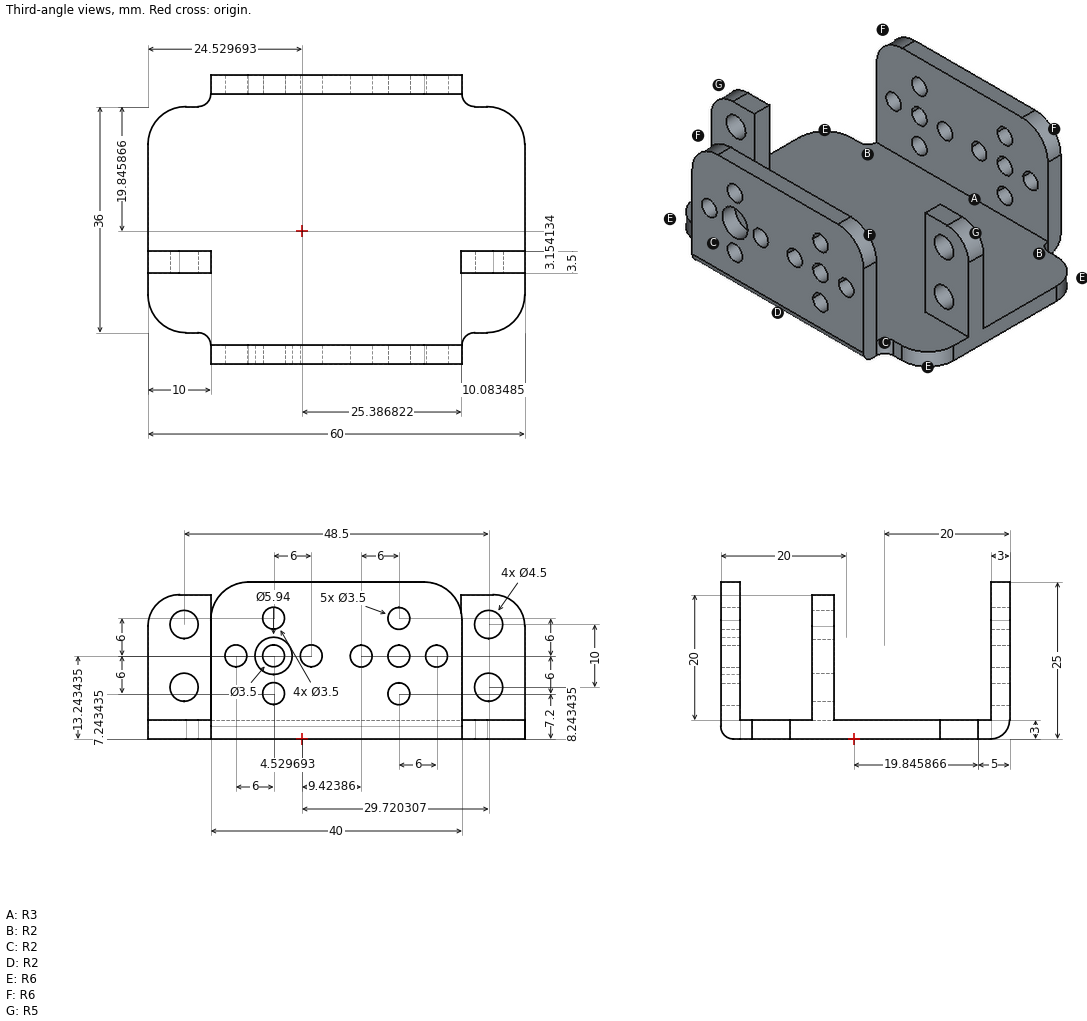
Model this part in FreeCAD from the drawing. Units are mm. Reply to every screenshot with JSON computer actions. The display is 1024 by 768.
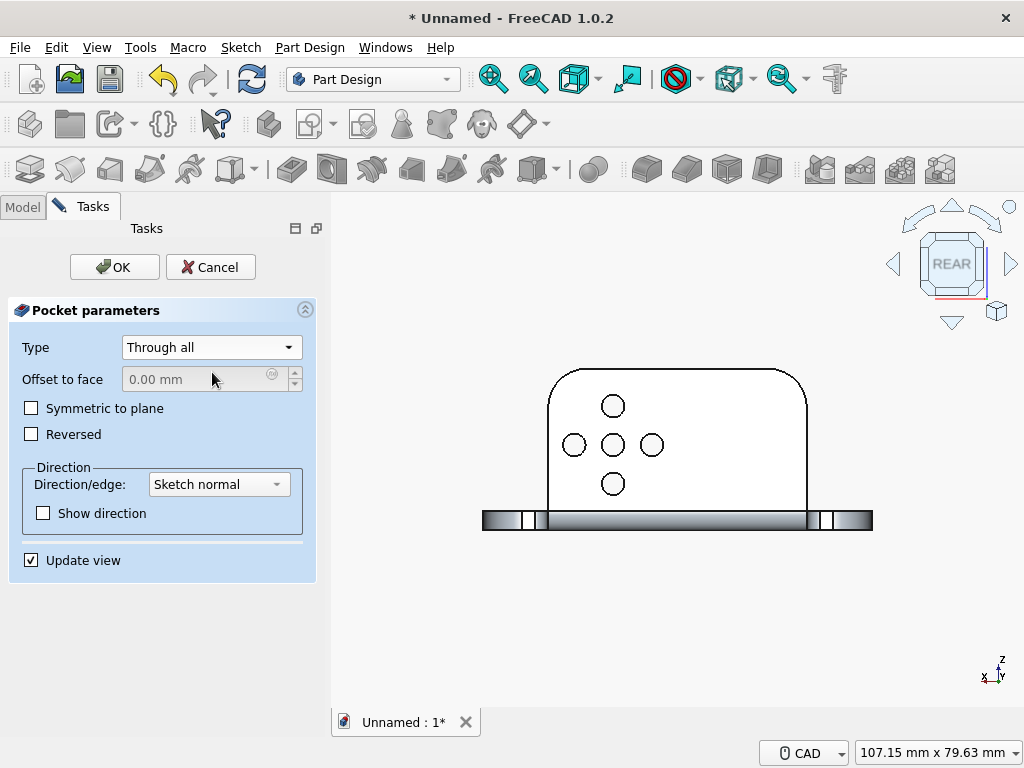
{"action": "left_click", "coordinate": [115, 267]}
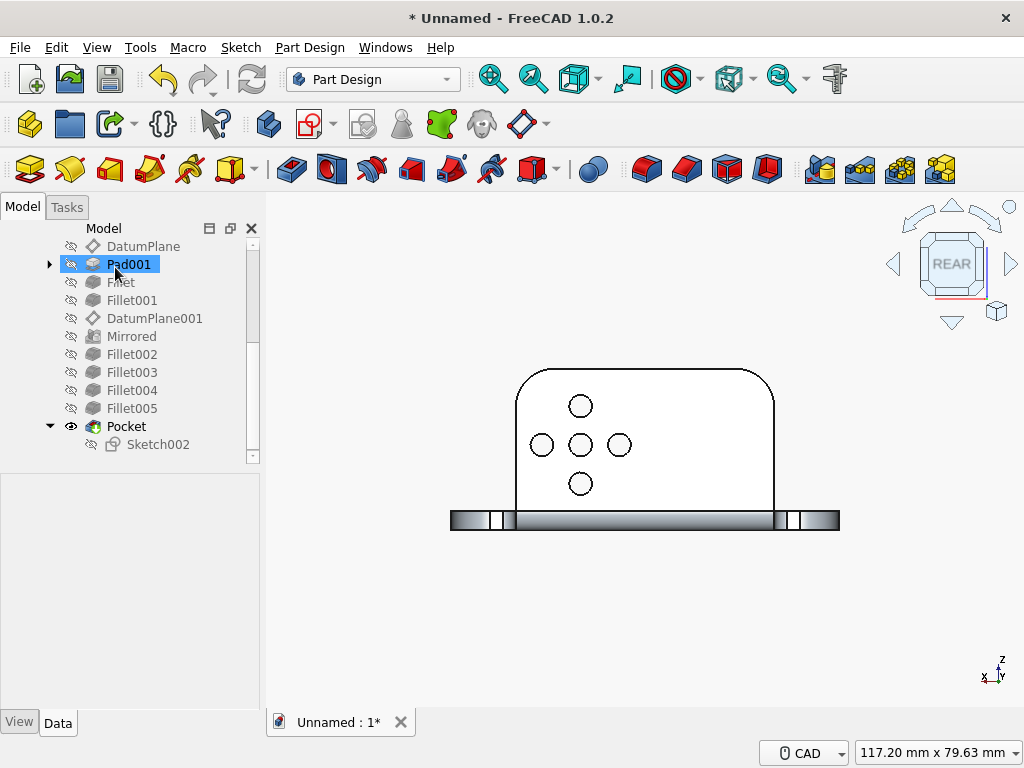
{"action": "key", "text": "0"}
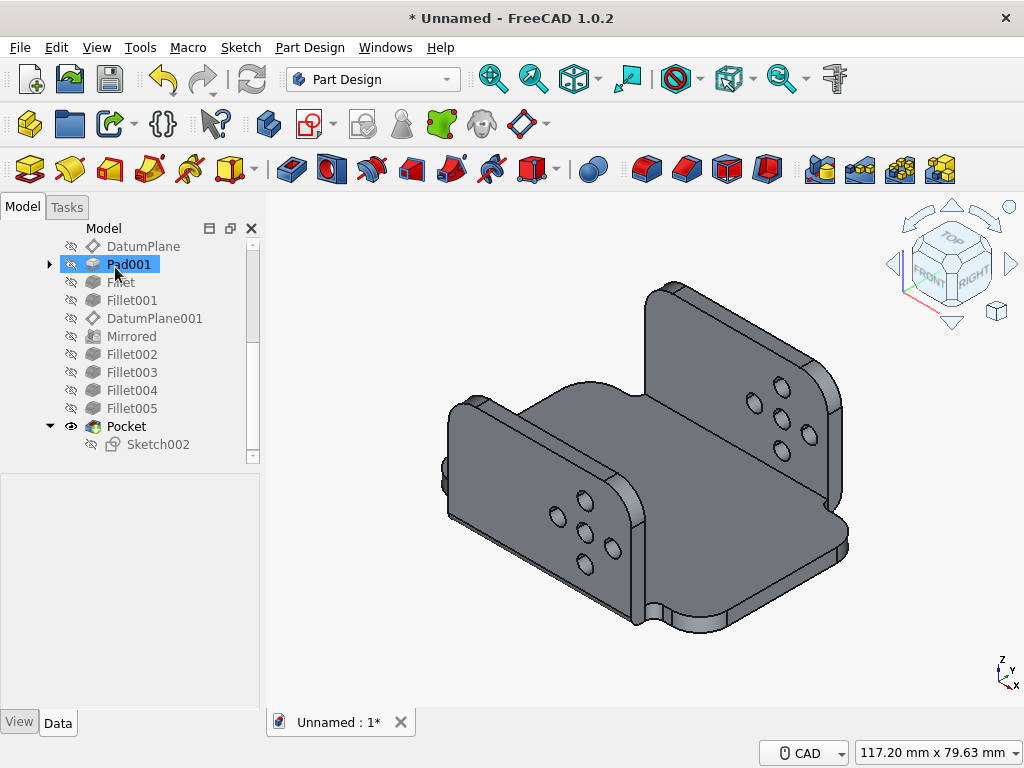
{"action": "left_click", "coordinate": [684, 521]}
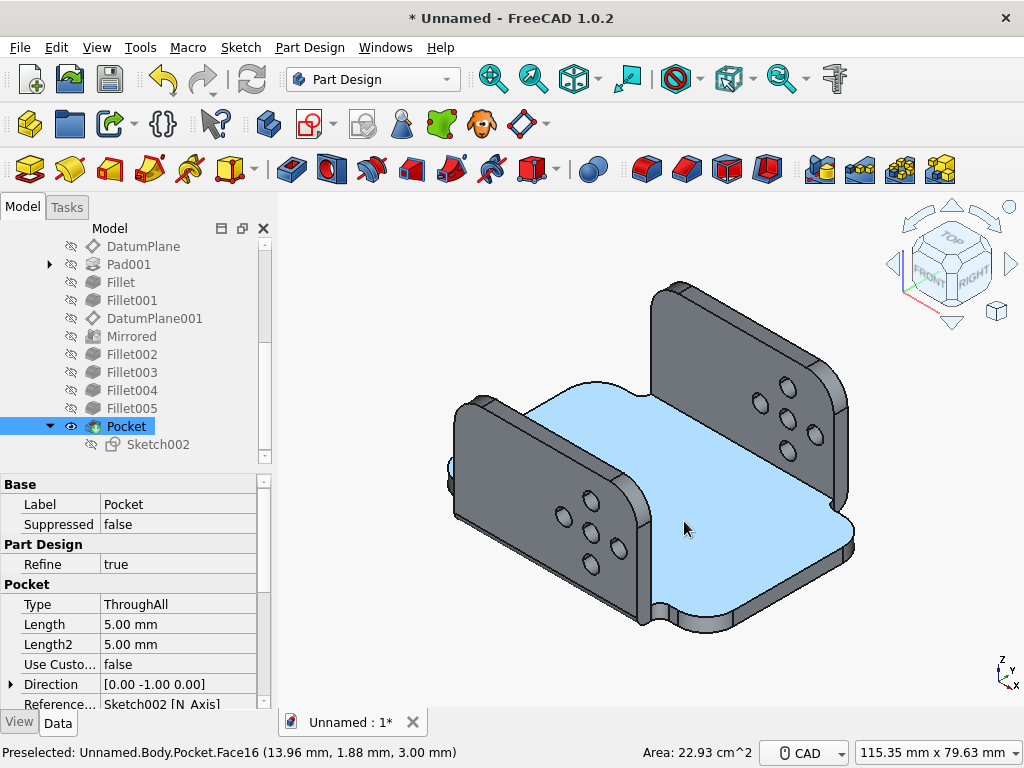
{"action": "left_click", "coordinate": [310, 124]}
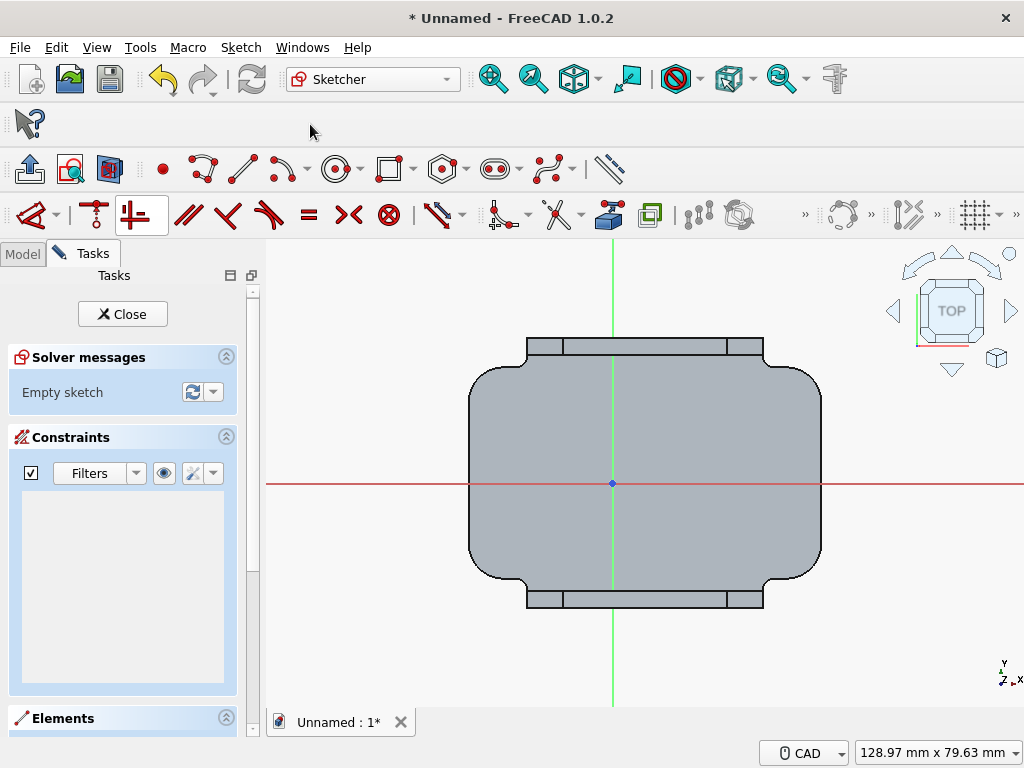
{"action": "left_click", "coordinate": [110, 170]}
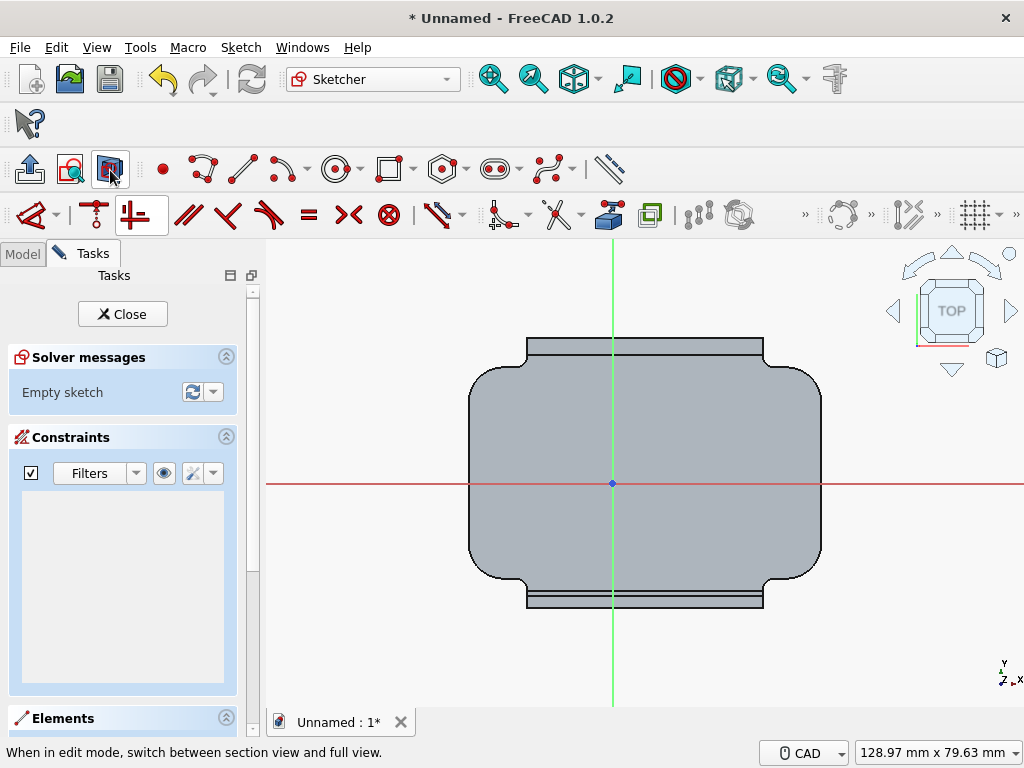
{"action": "left_click", "coordinate": [390, 170]}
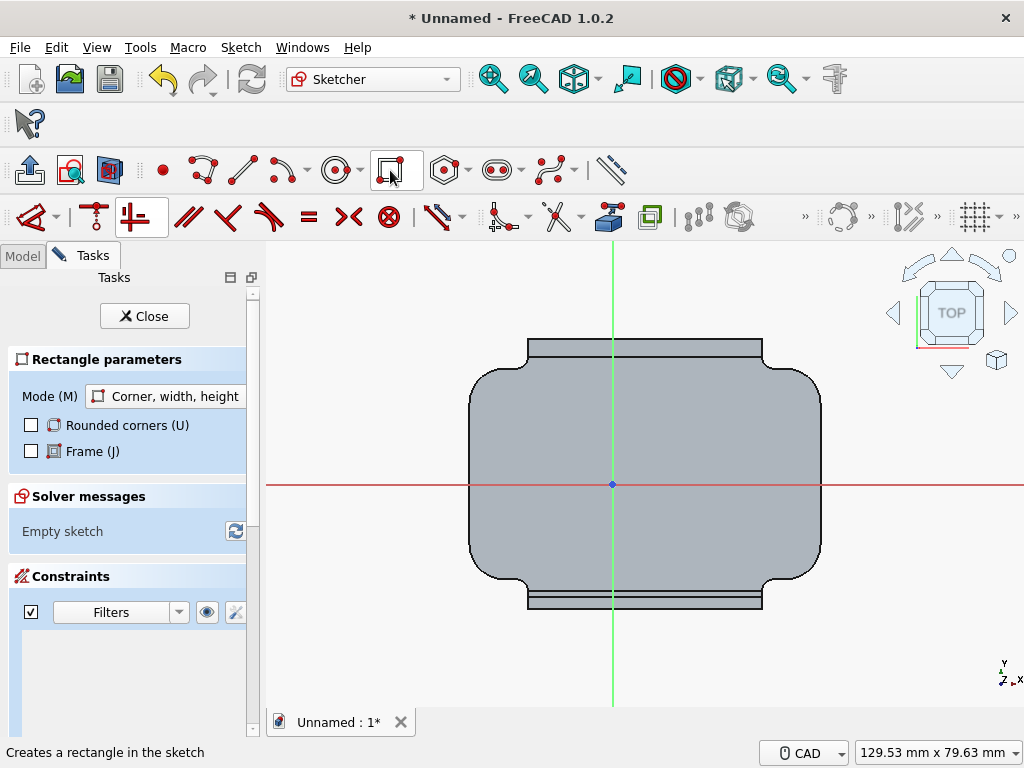
{"action": "left_click", "coordinate": [762, 503]}
{"action": "left_click", "coordinate": [821, 524]}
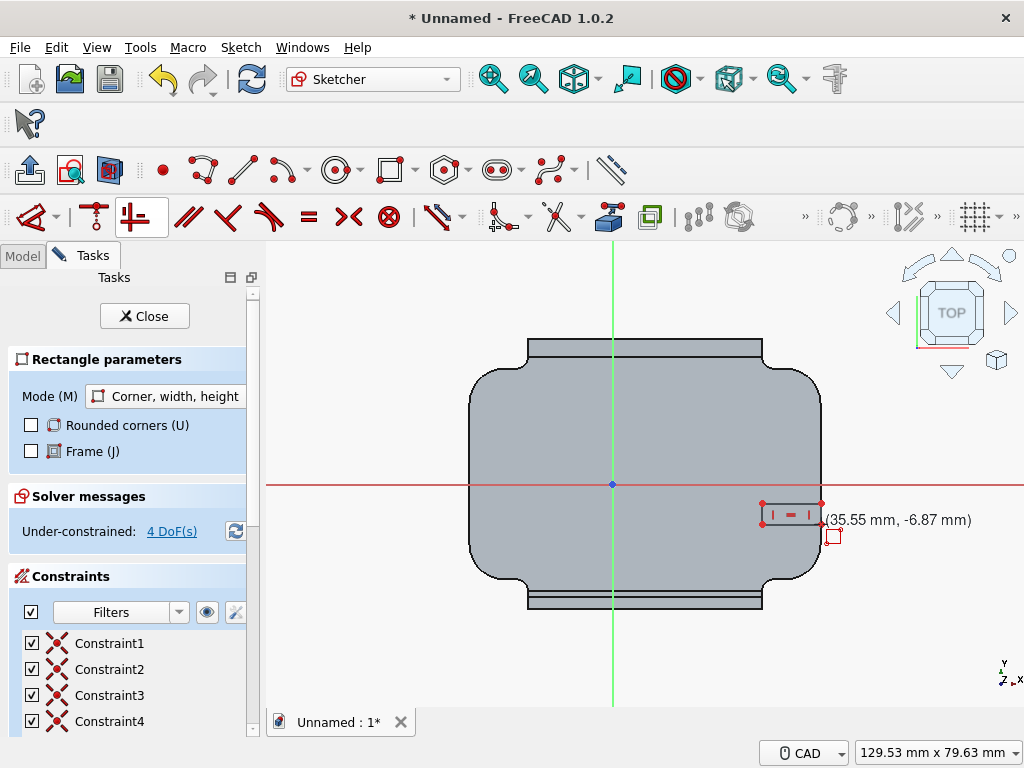
{"action": "left_click", "coordinate": [469, 503]}
{"action": "left_click", "coordinate": [528, 524]}
{"action": "key", "text": "Escape"}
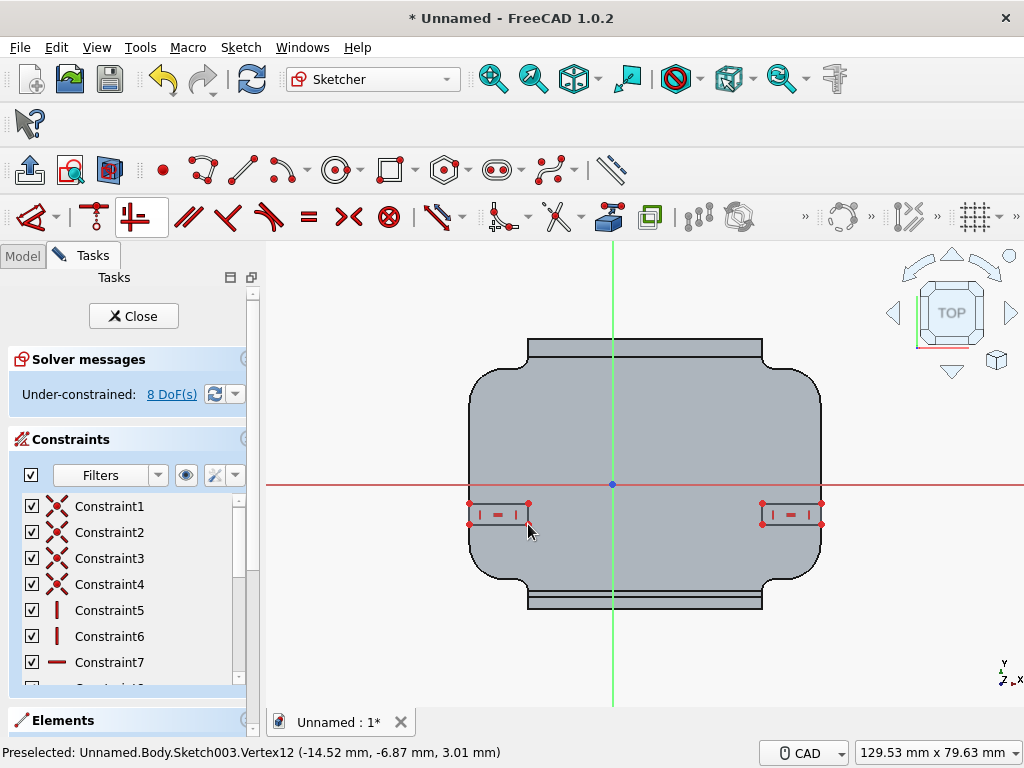
{"action": "left_click", "coordinate": [32, 218]}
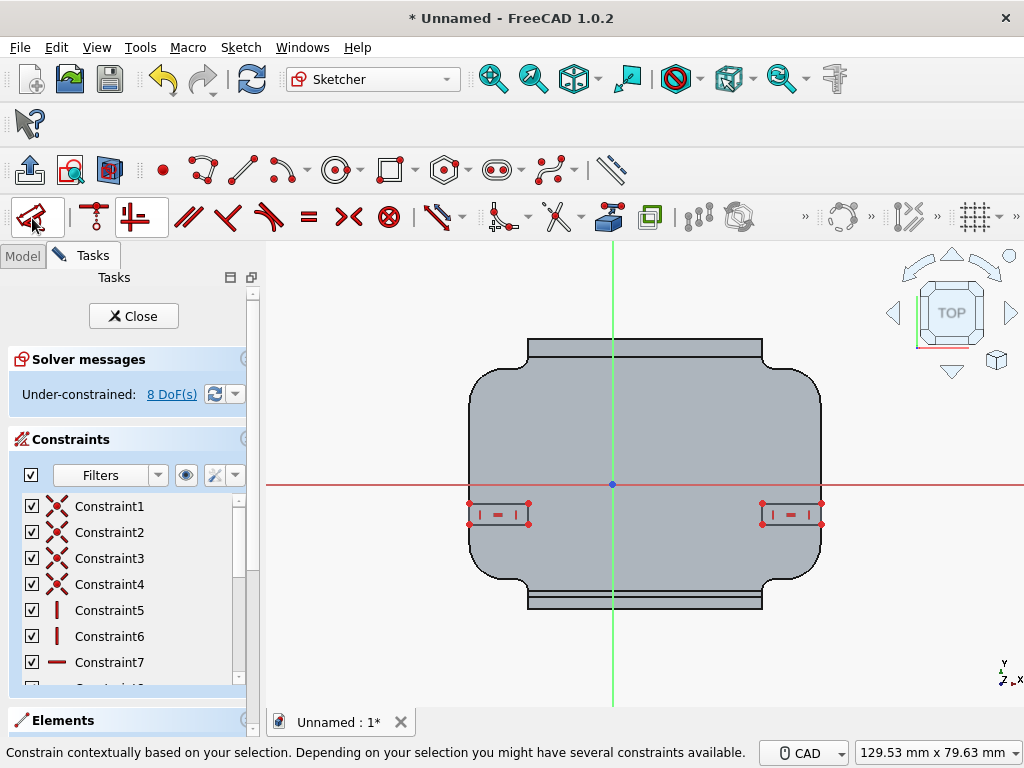
{"action": "left_click", "coordinate": [487, 525]}
{"action": "left_click", "coordinate": [499, 559]}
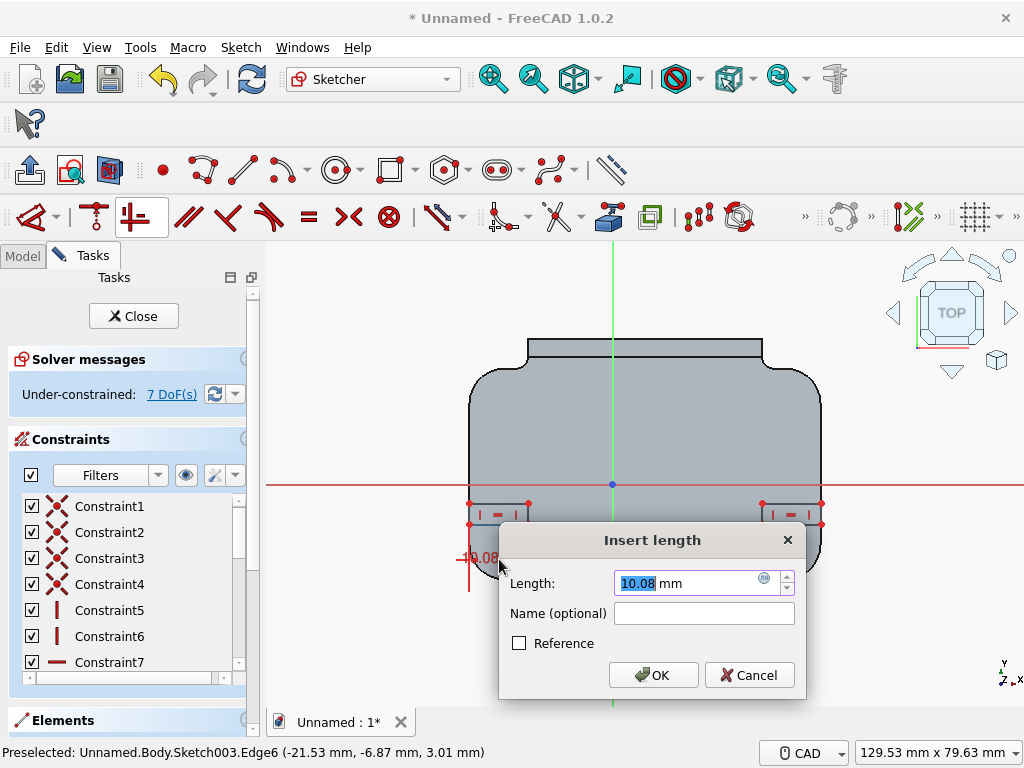
{"action": "type", "text": "10"}
{"action": "key", "text": "Return"}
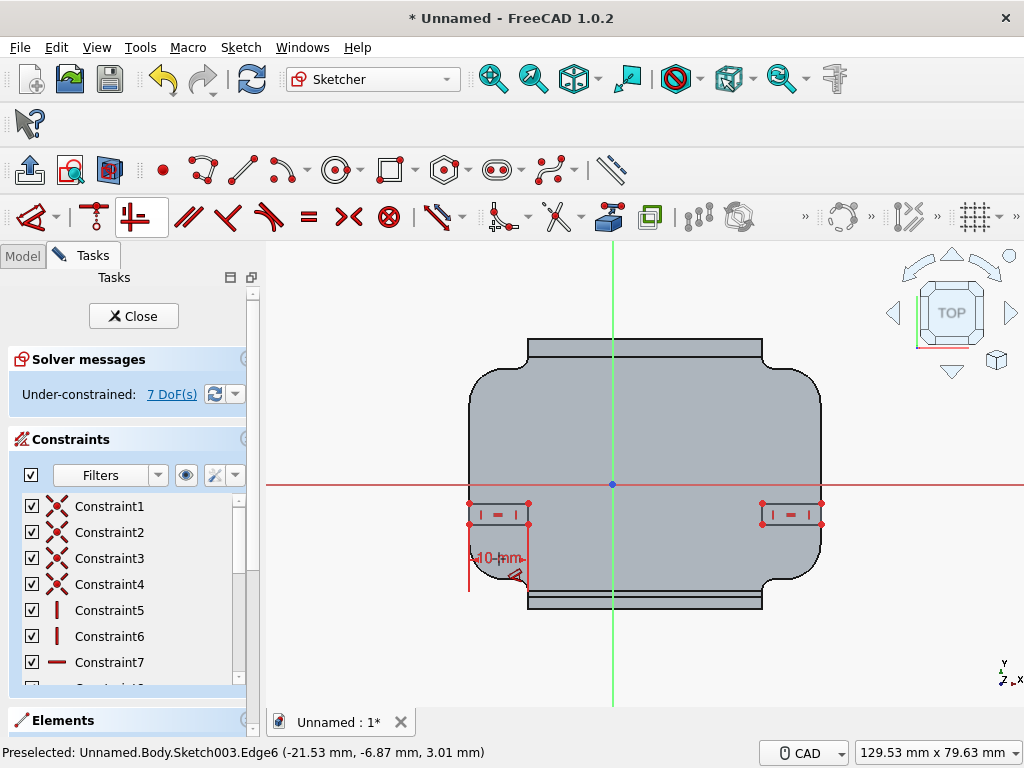
{"action": "scroll", "coordinate": [762, 515], "scroll_direction": "up", "scroll_amount": 4}